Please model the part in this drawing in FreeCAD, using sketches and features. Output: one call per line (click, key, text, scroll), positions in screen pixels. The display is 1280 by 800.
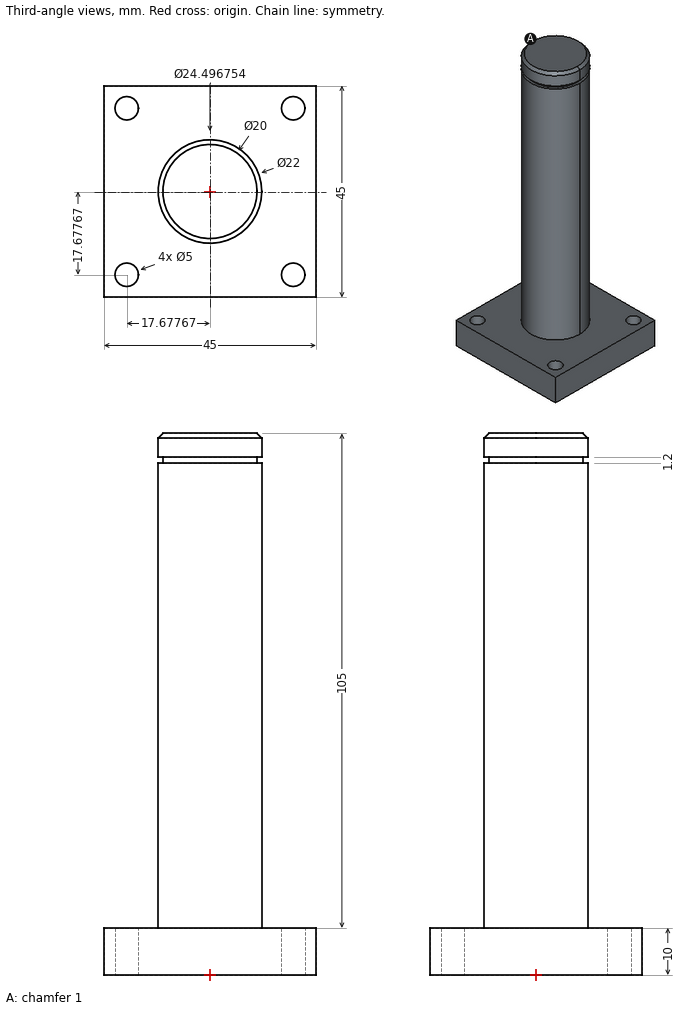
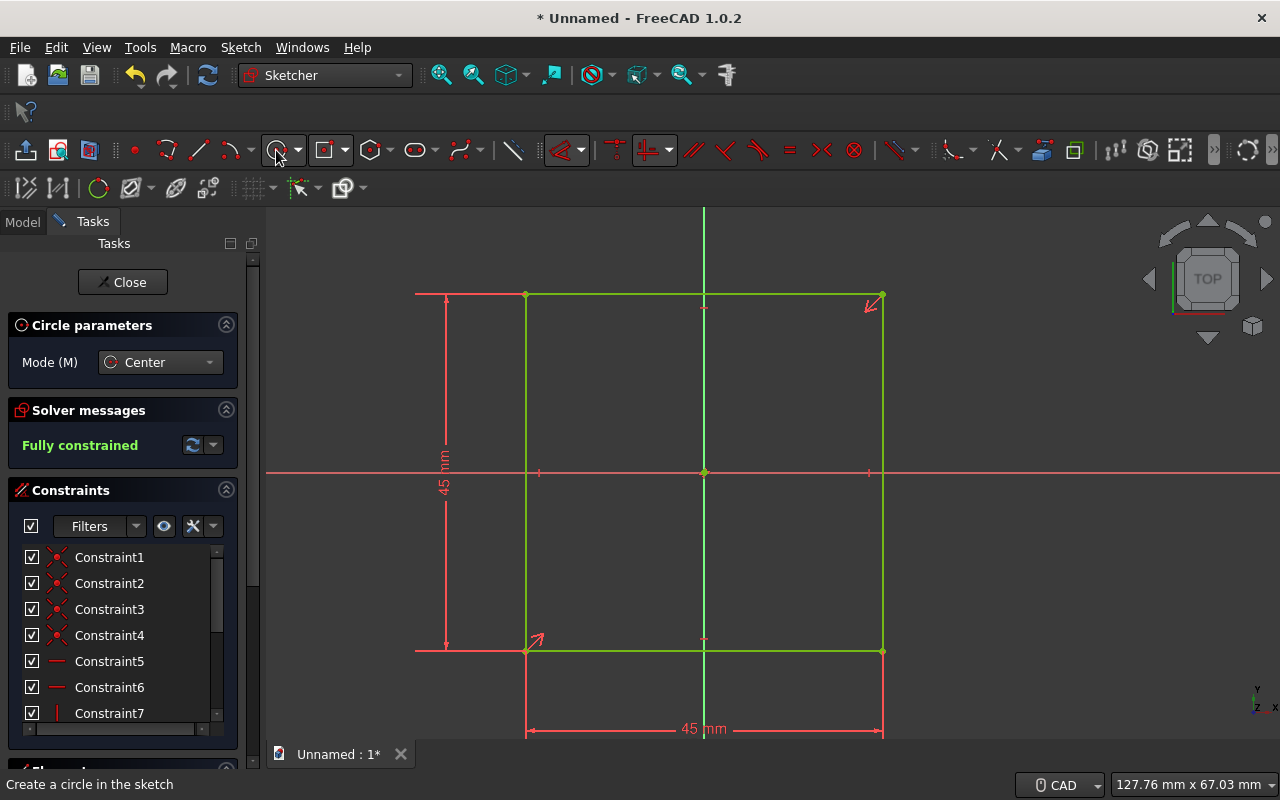
click(564, 613)
move(578, 599)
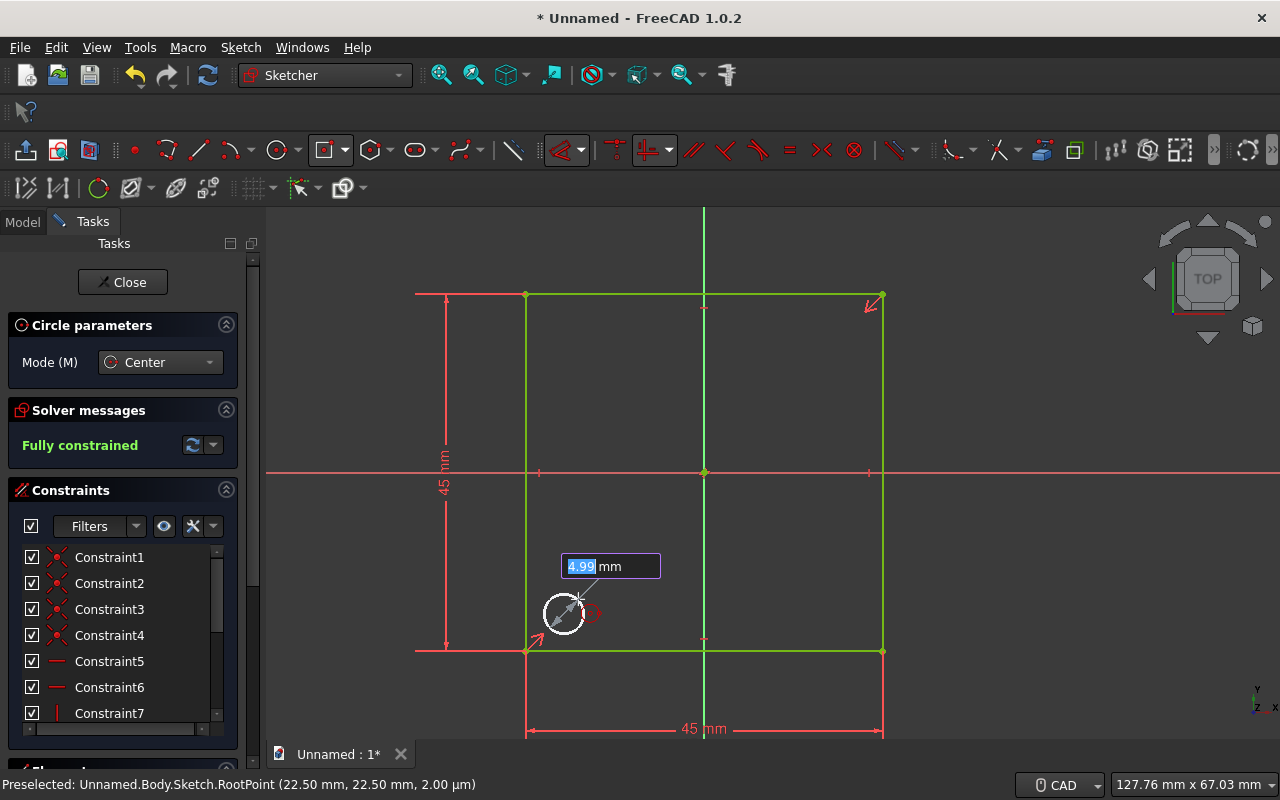
text(5)
key(Return)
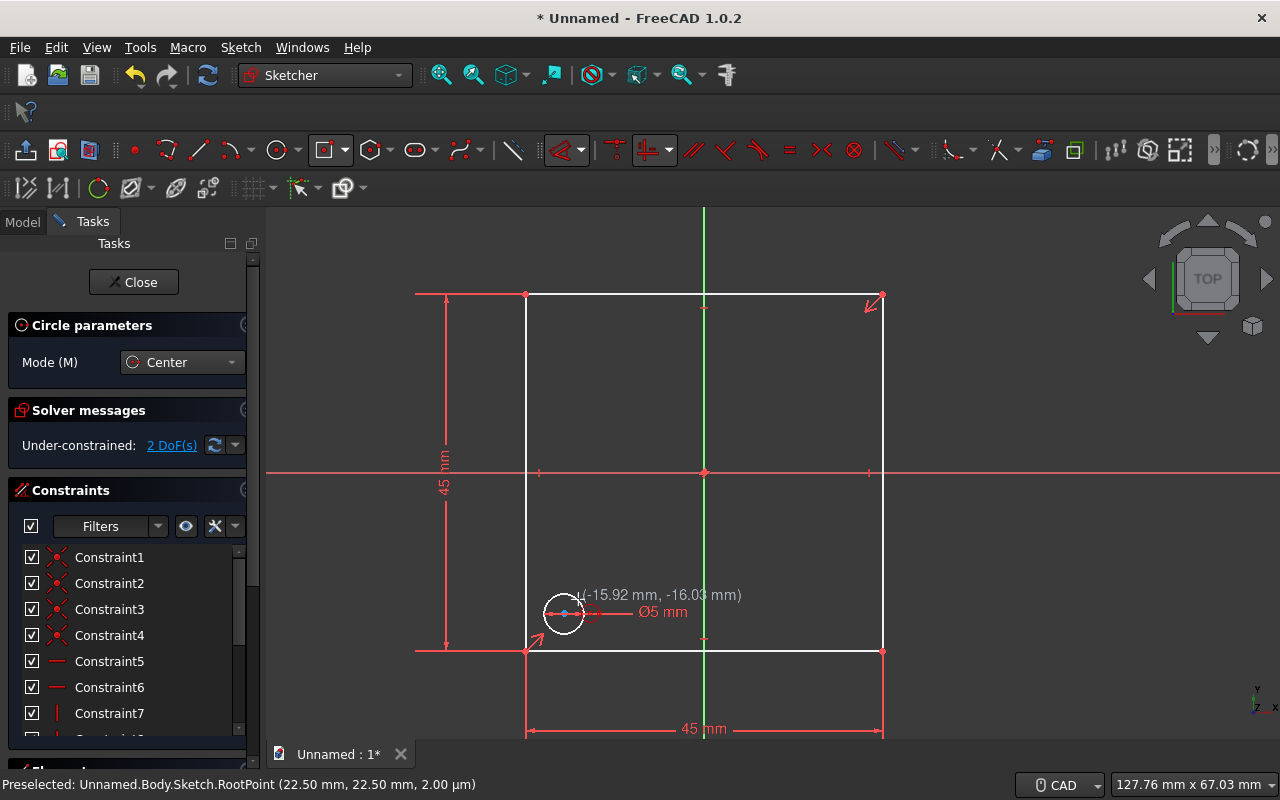
click(845, 613)
move(859, 599)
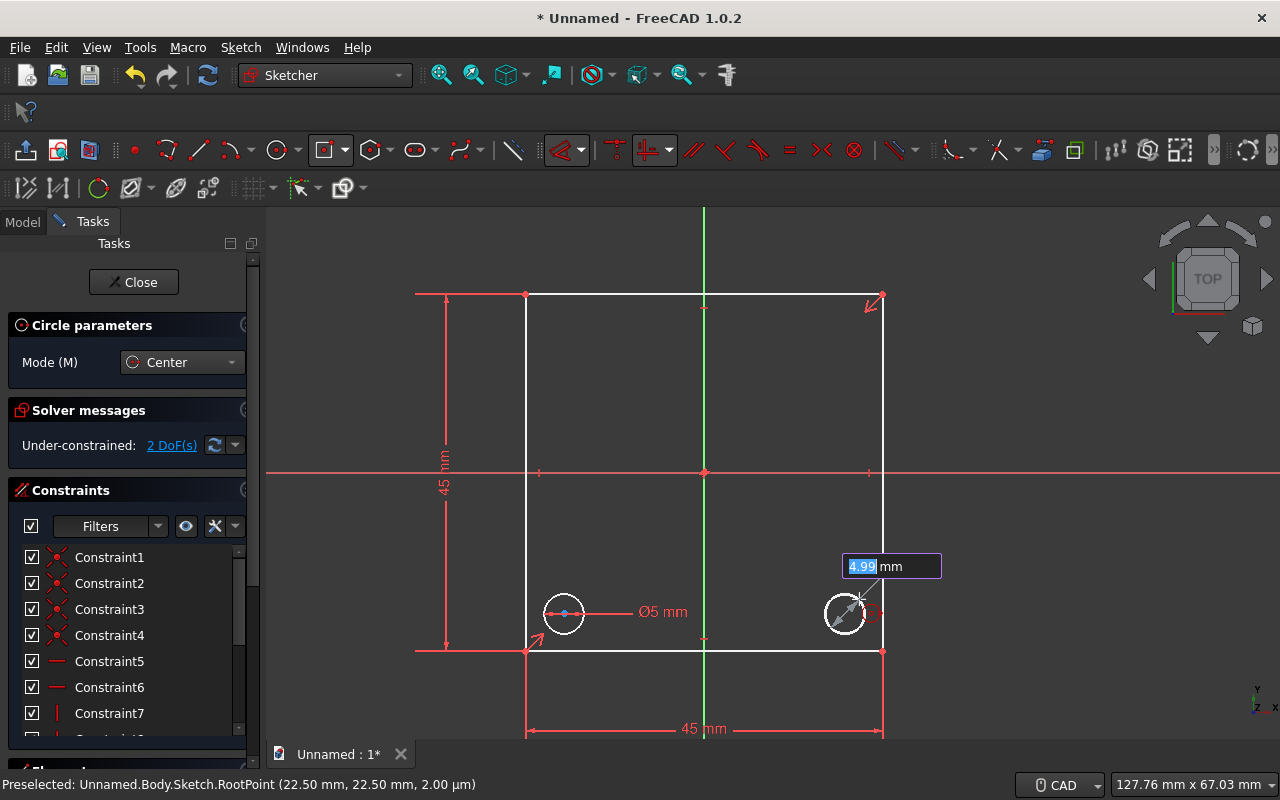
text(5)
key(Return)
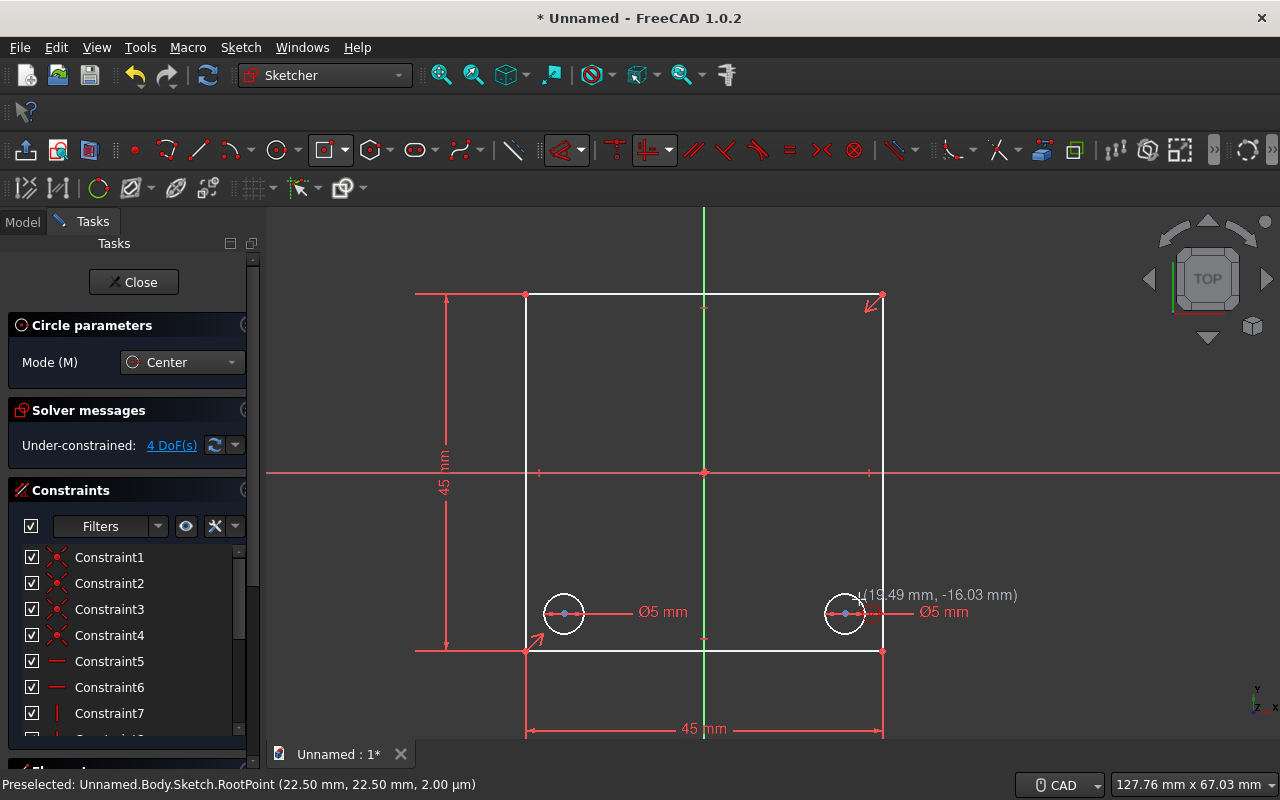
click(564, 332)
move(578, 318)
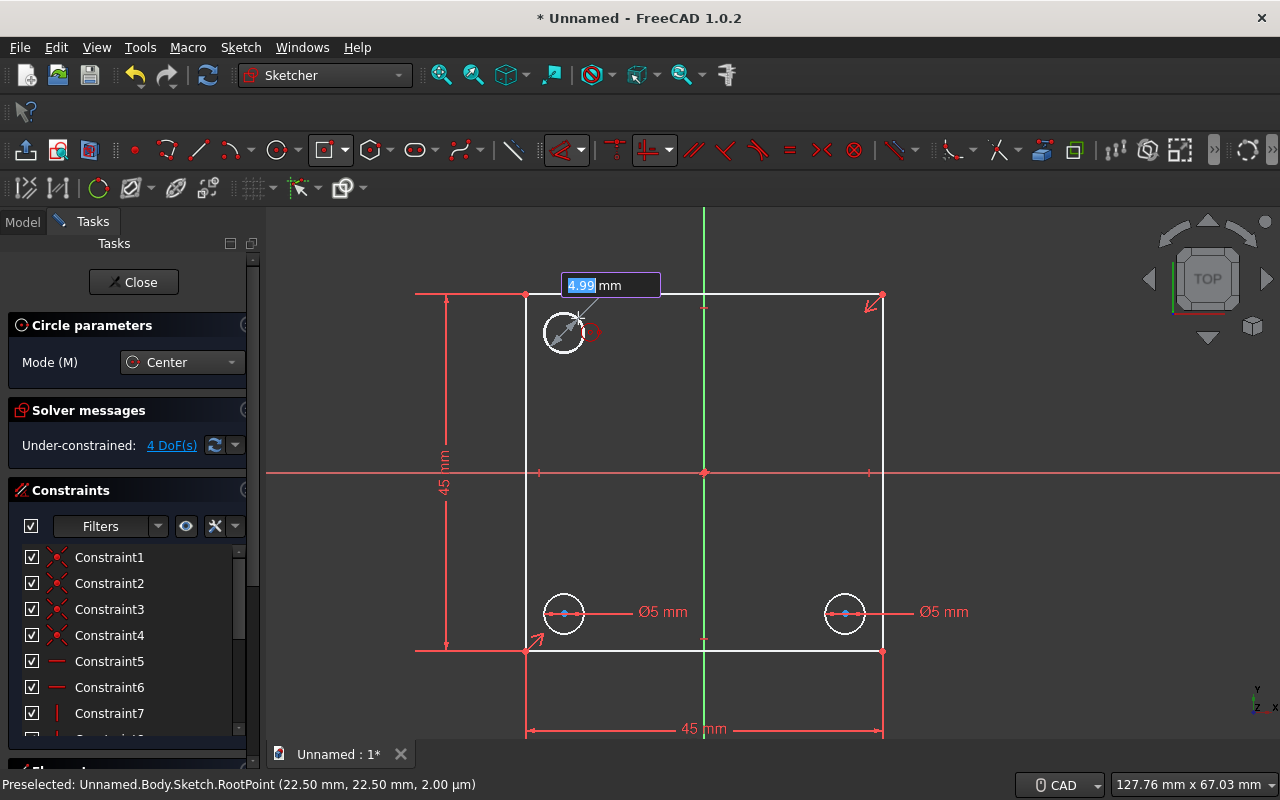
text(5)
key(Return)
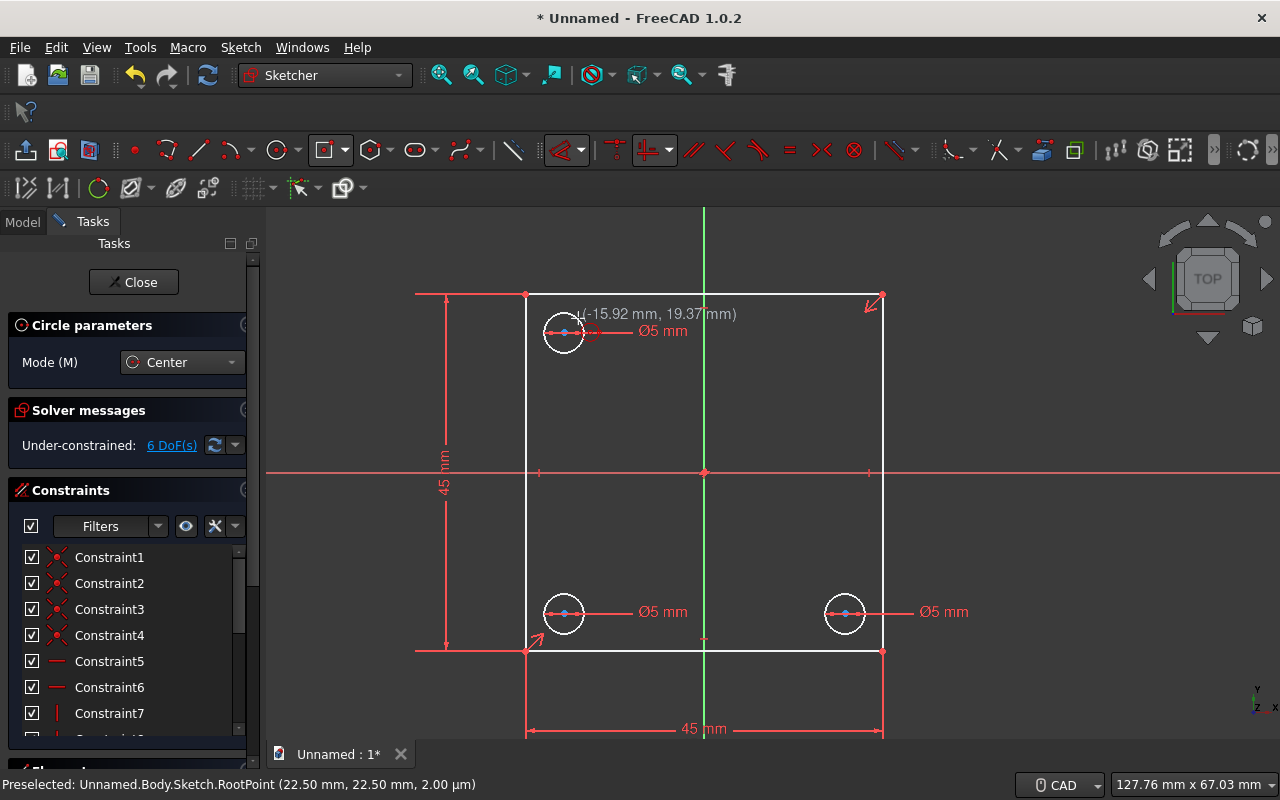
click(845, 332)
move(859, 318)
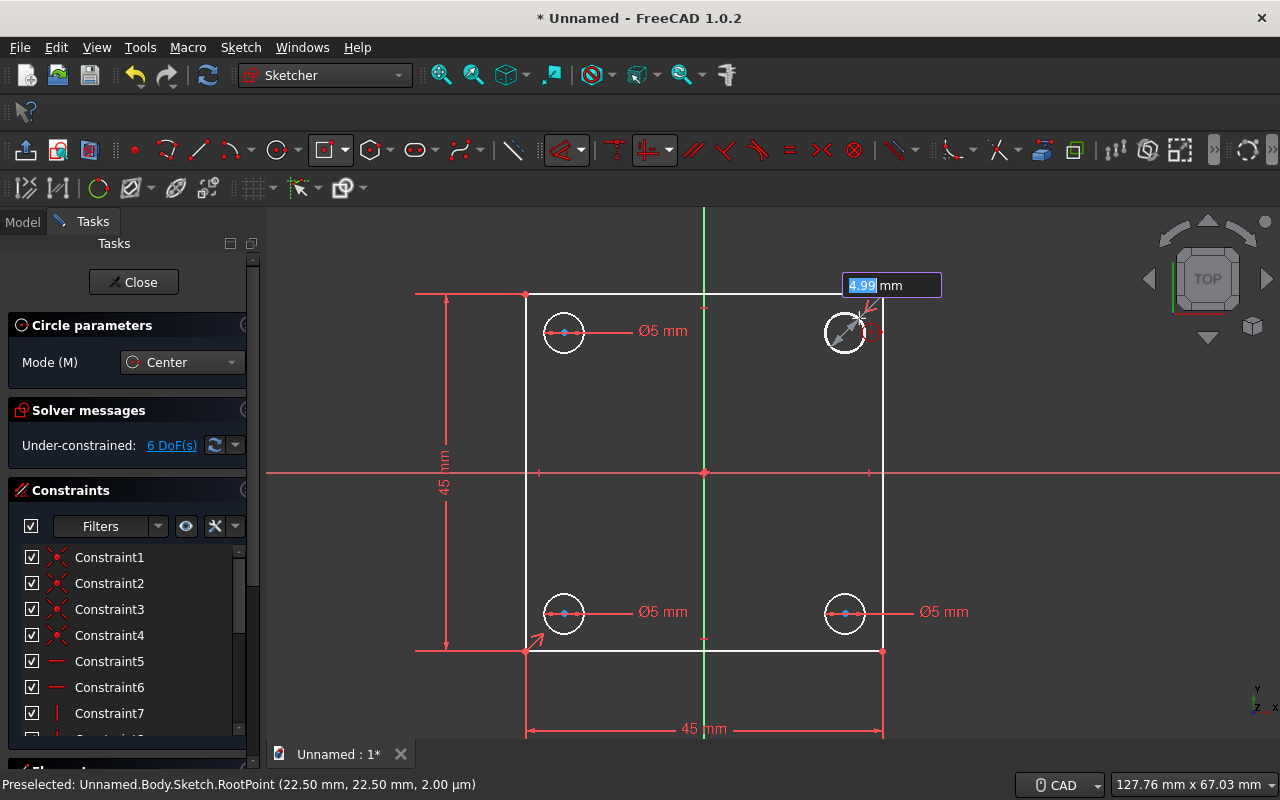
text(5)
key(Return)
key(Escape)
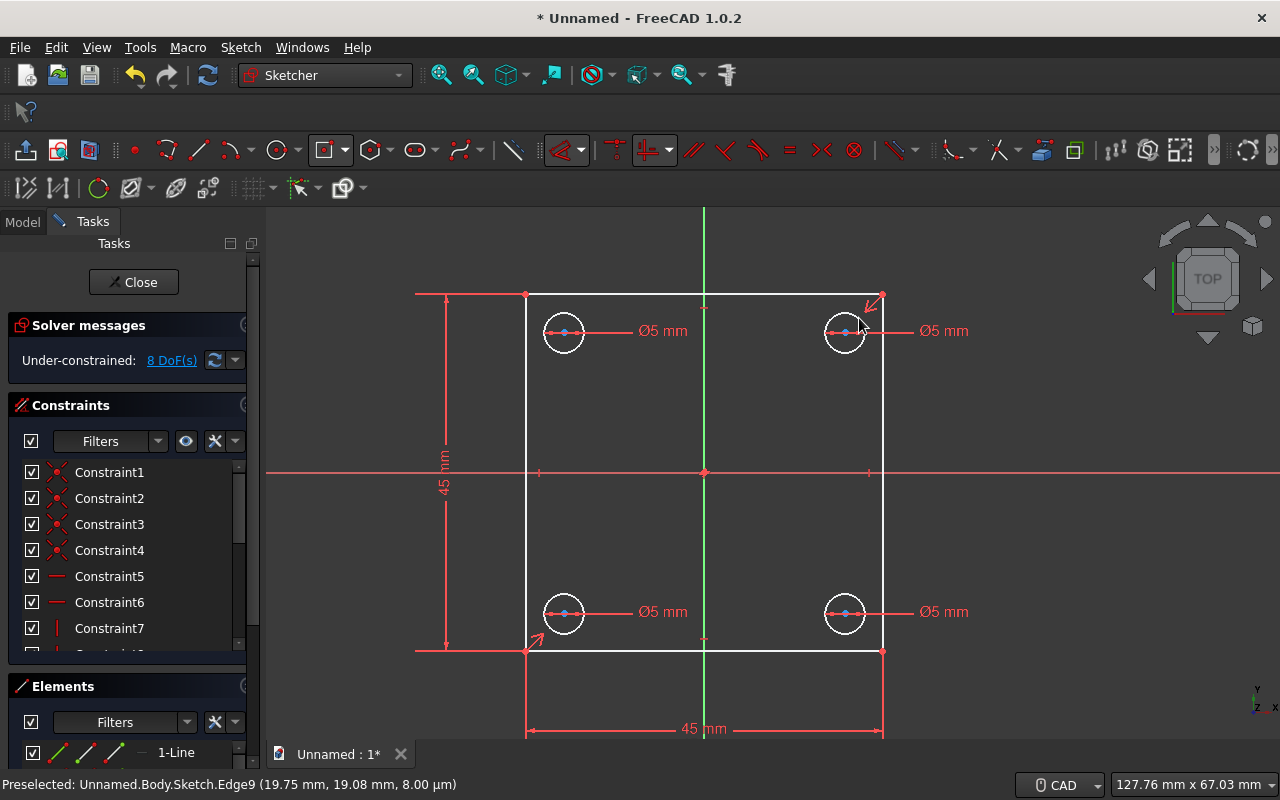
click(564, 614)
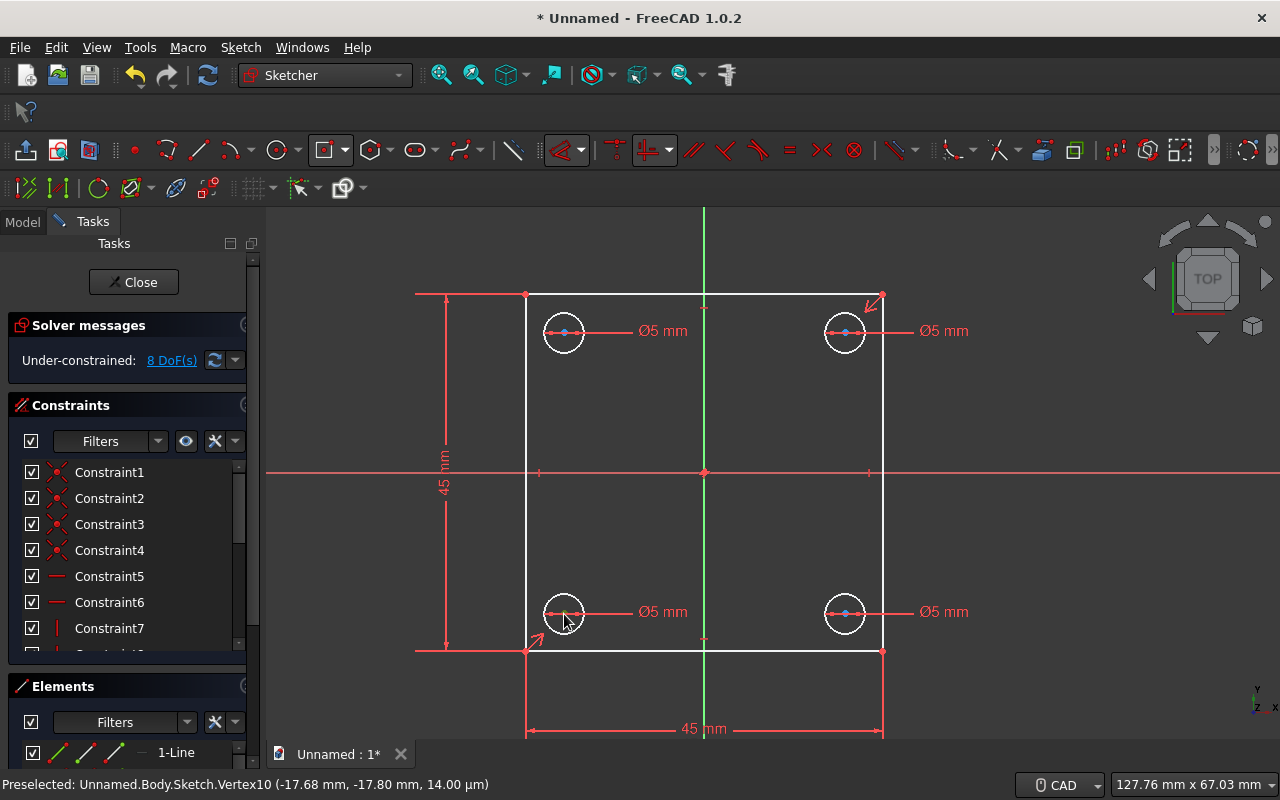
click(845, 614)